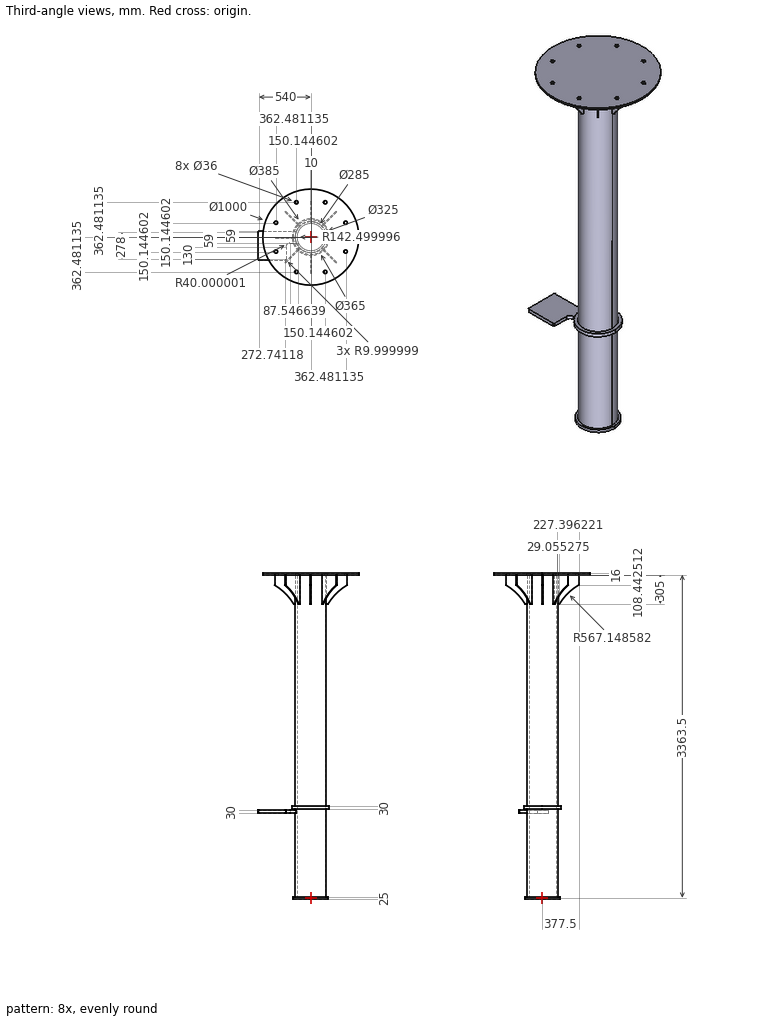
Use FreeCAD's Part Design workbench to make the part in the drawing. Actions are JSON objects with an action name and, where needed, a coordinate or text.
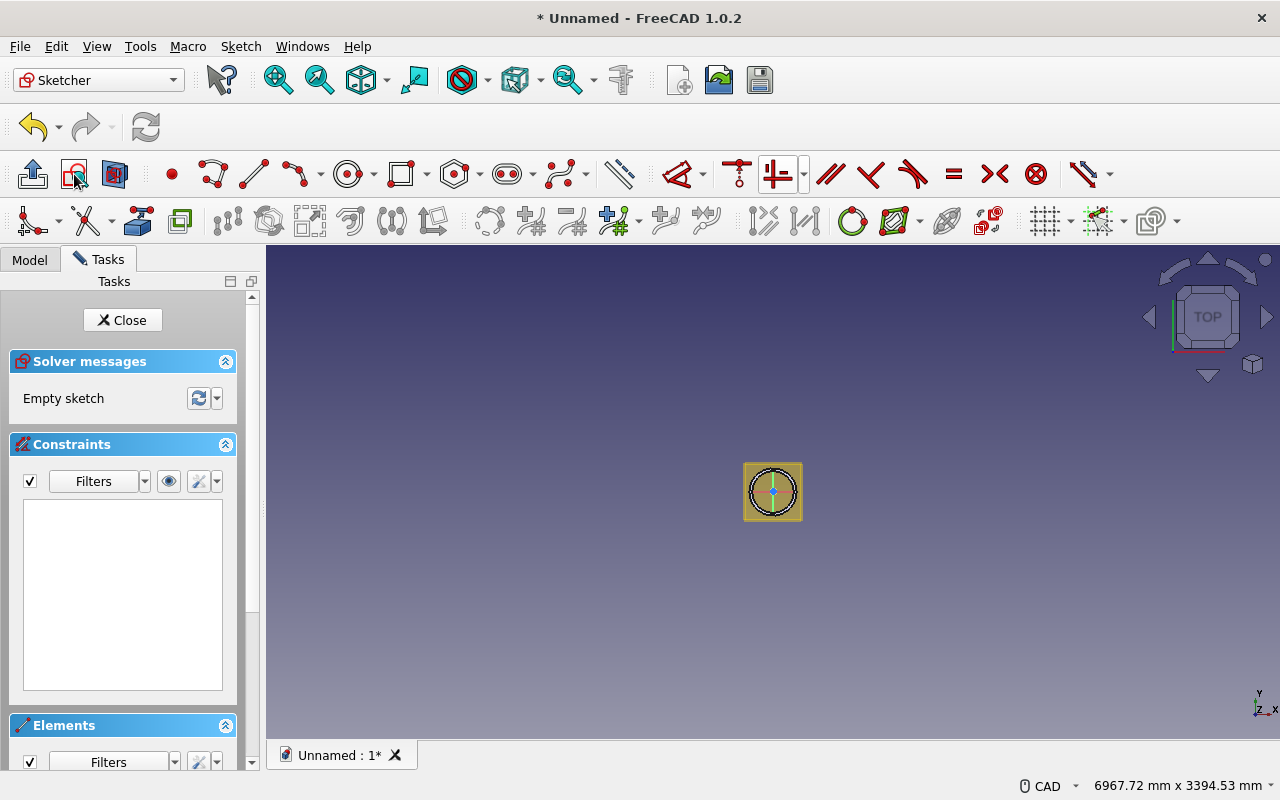
{"action": "key", "text": "q s"}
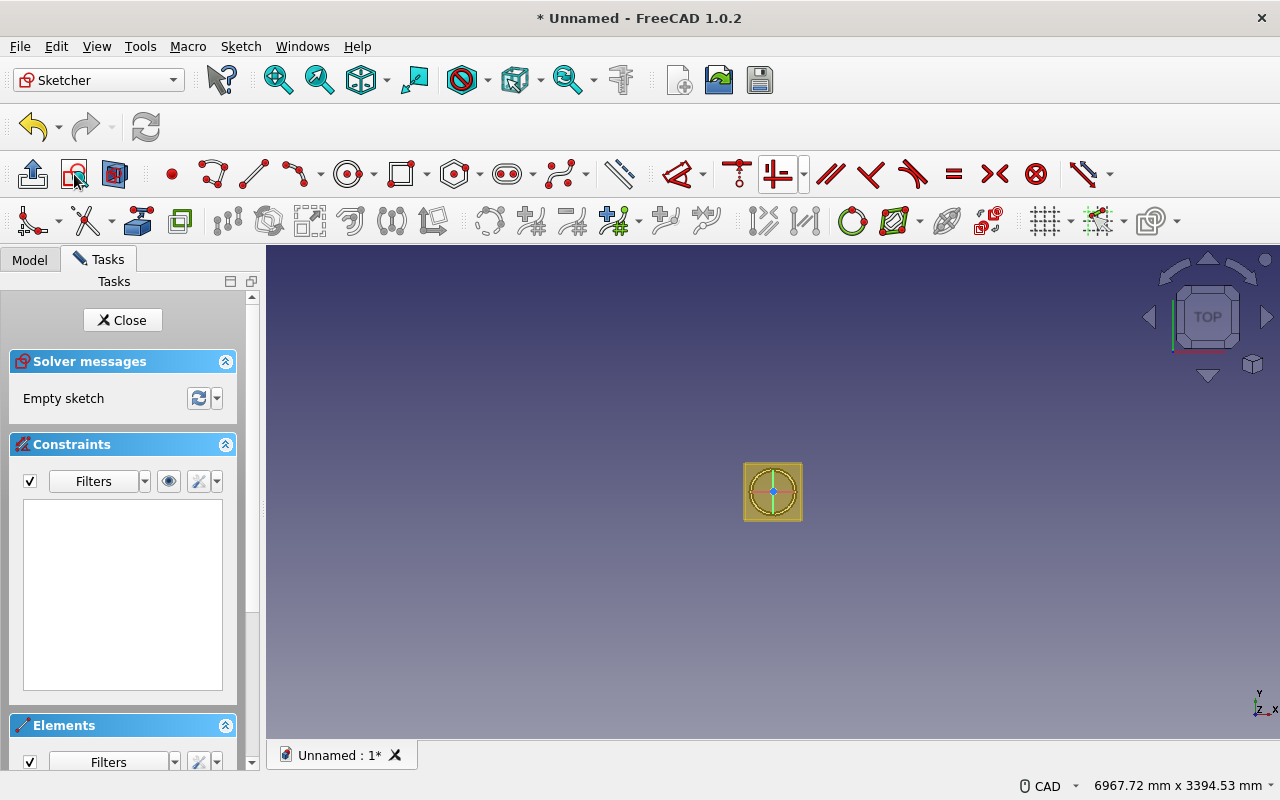
{"action": "scroll", "coordinate": [787, 492], "scroll_direction": "up", "scroll_amount": 9}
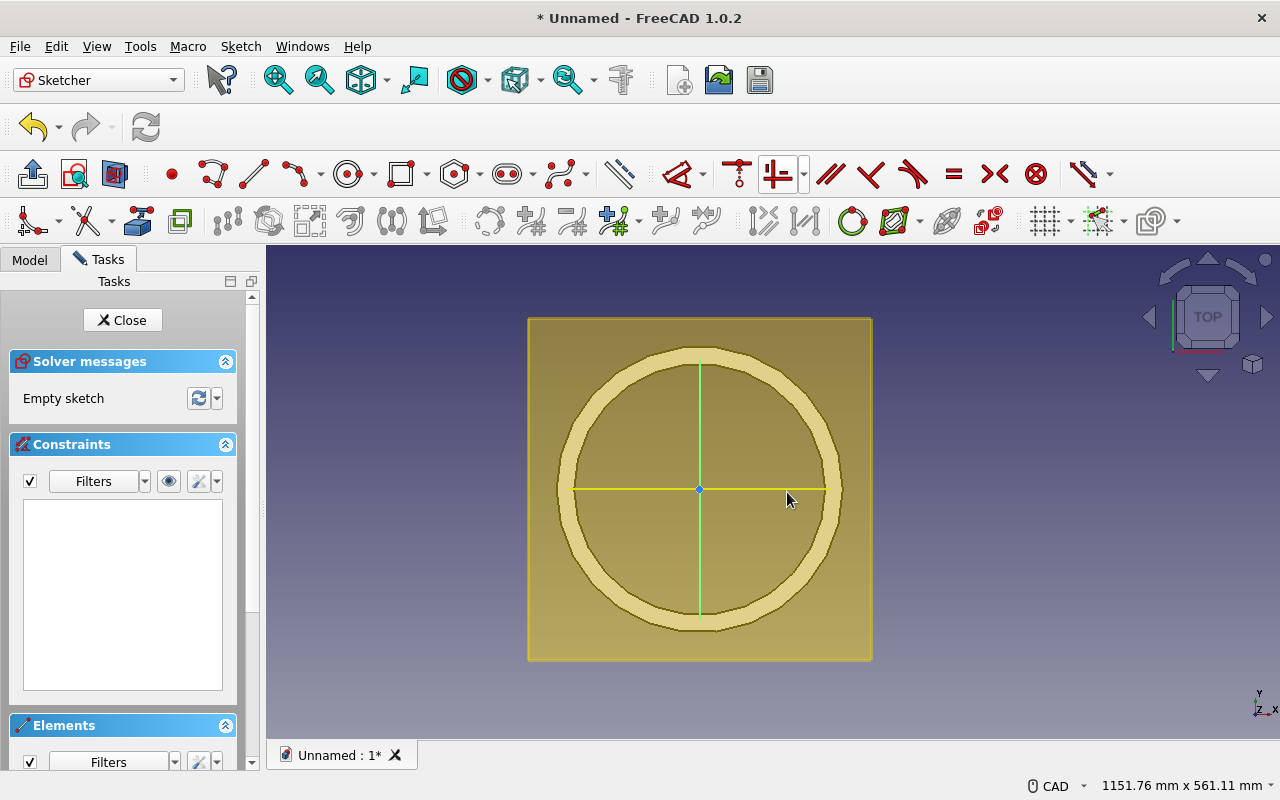
{"action": "left_click", "coordinate": [348, 174]}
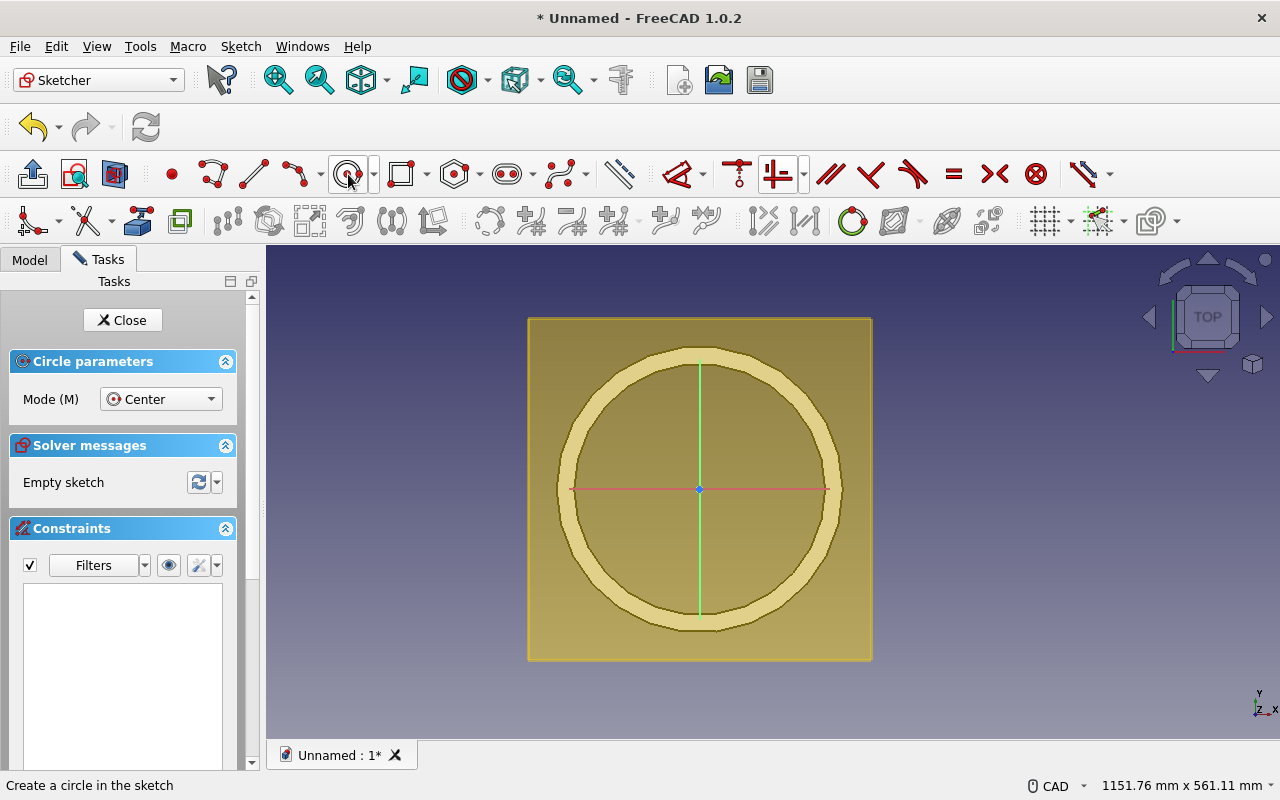
{"action": "left_click", "coordinate": [700, 489]}
{"action": "left_click", "coordinate": [820, 370]}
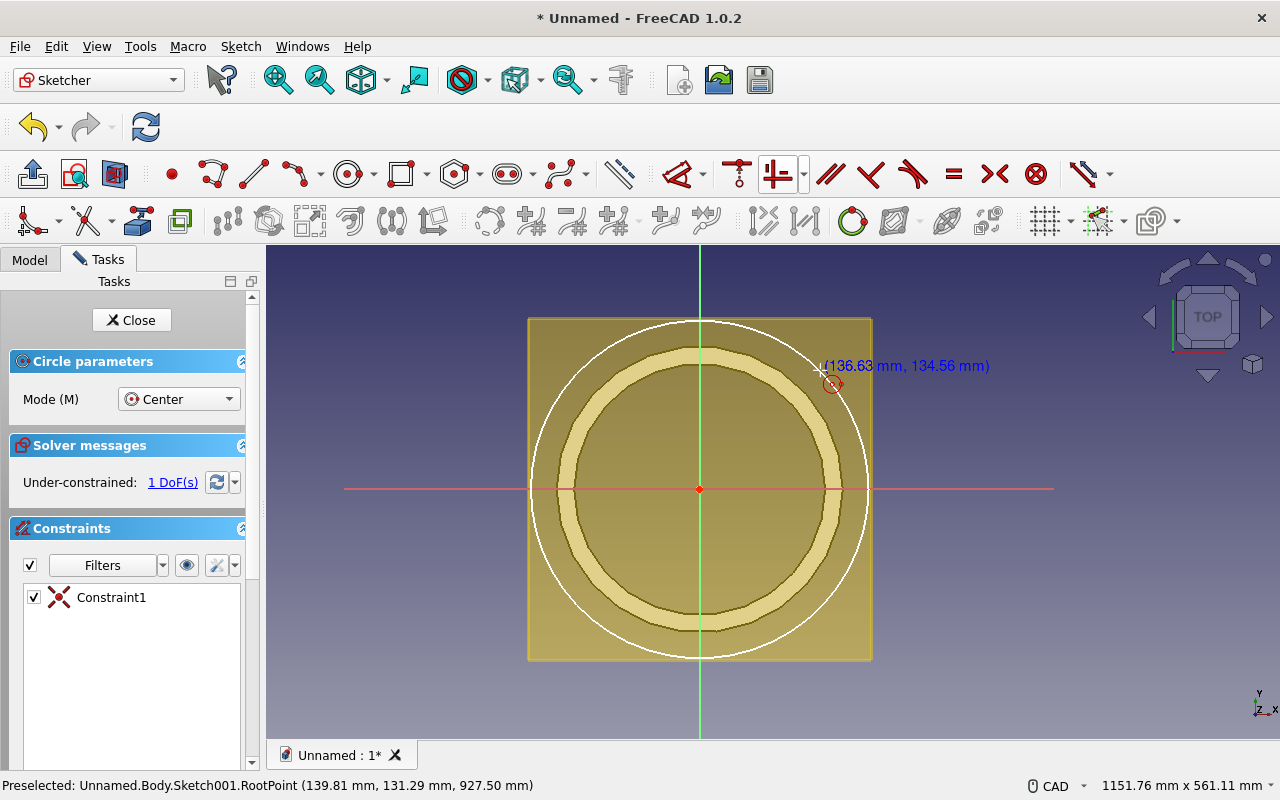
{"action": "left_click", "coordinate": [700, 489]}
{"action": "left_click", "coordinate": [801, 388]}
{"action": "key", "text": "Escape"}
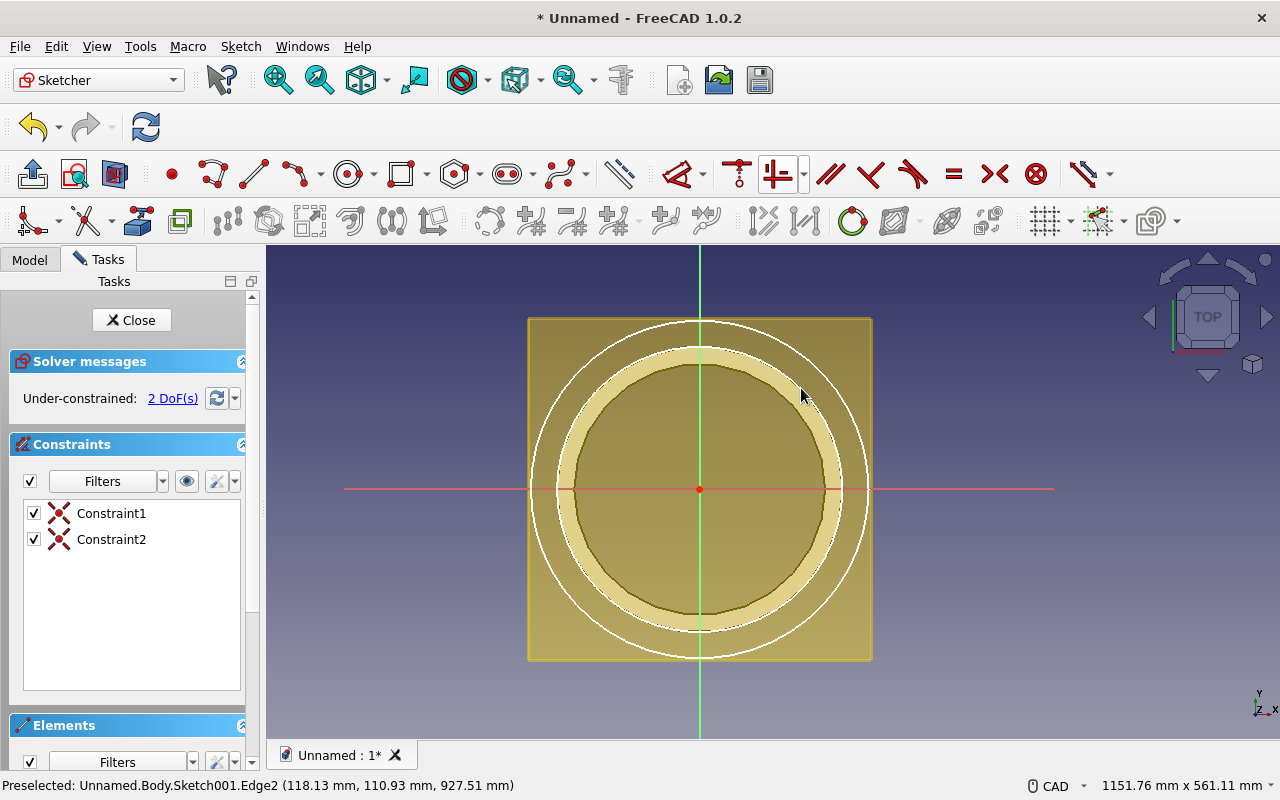
{"action": "left_click", "coordinate": [819, 370]}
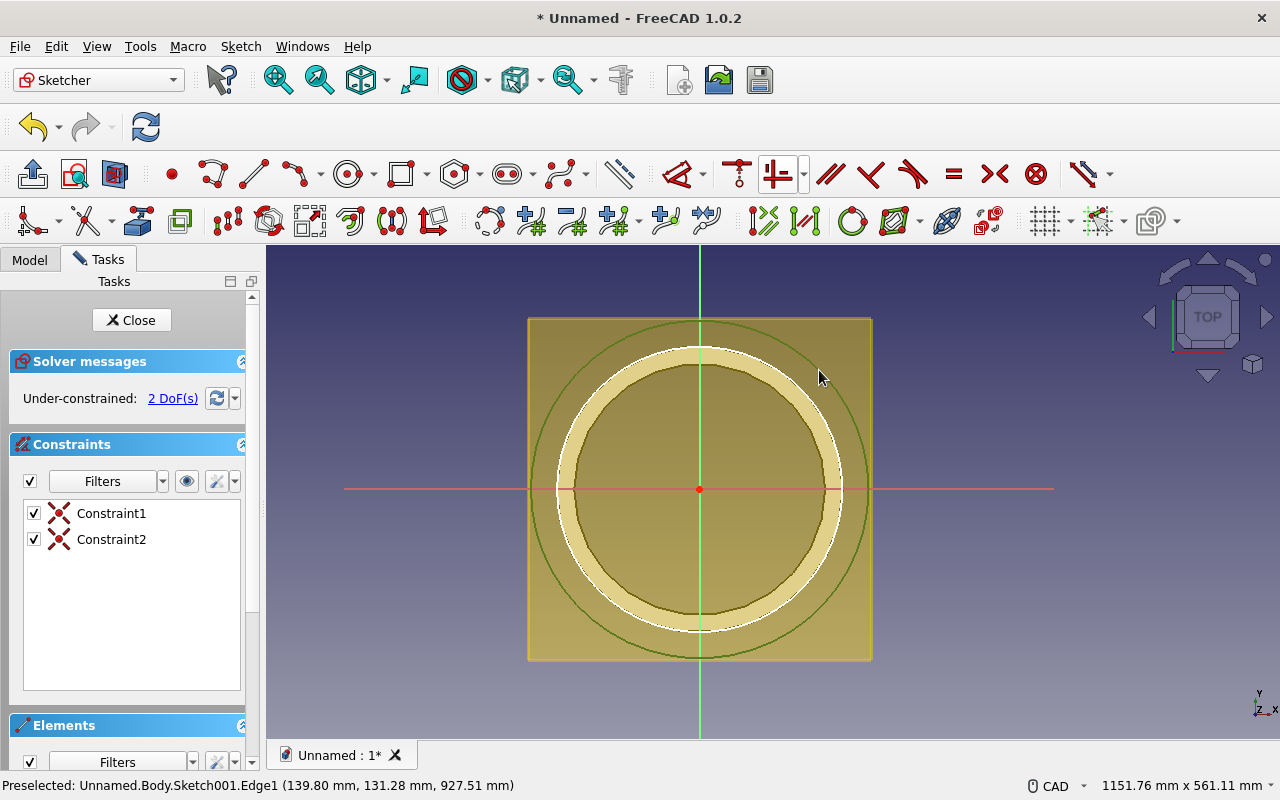
{"action": "key", "text": "k o"}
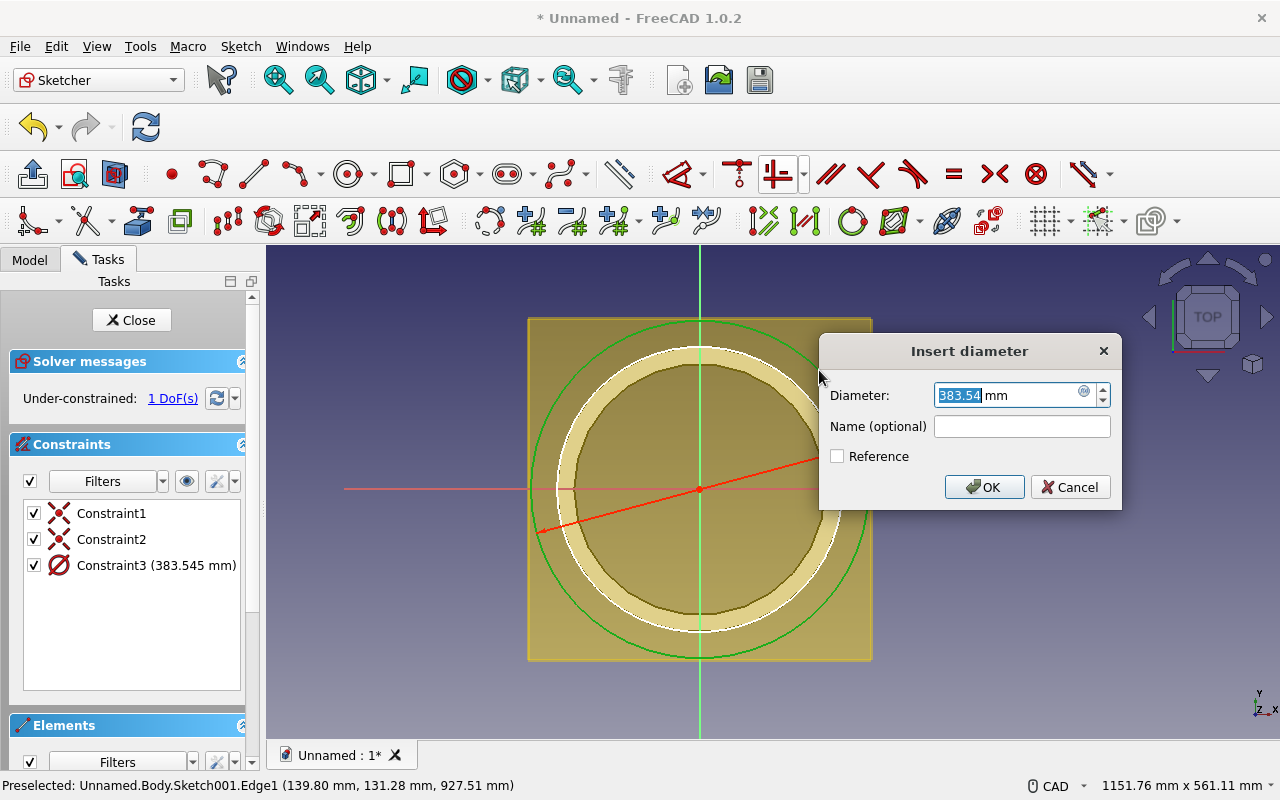
{"action": "type", "text": "385"}
{"action": "key", "text": "Return"}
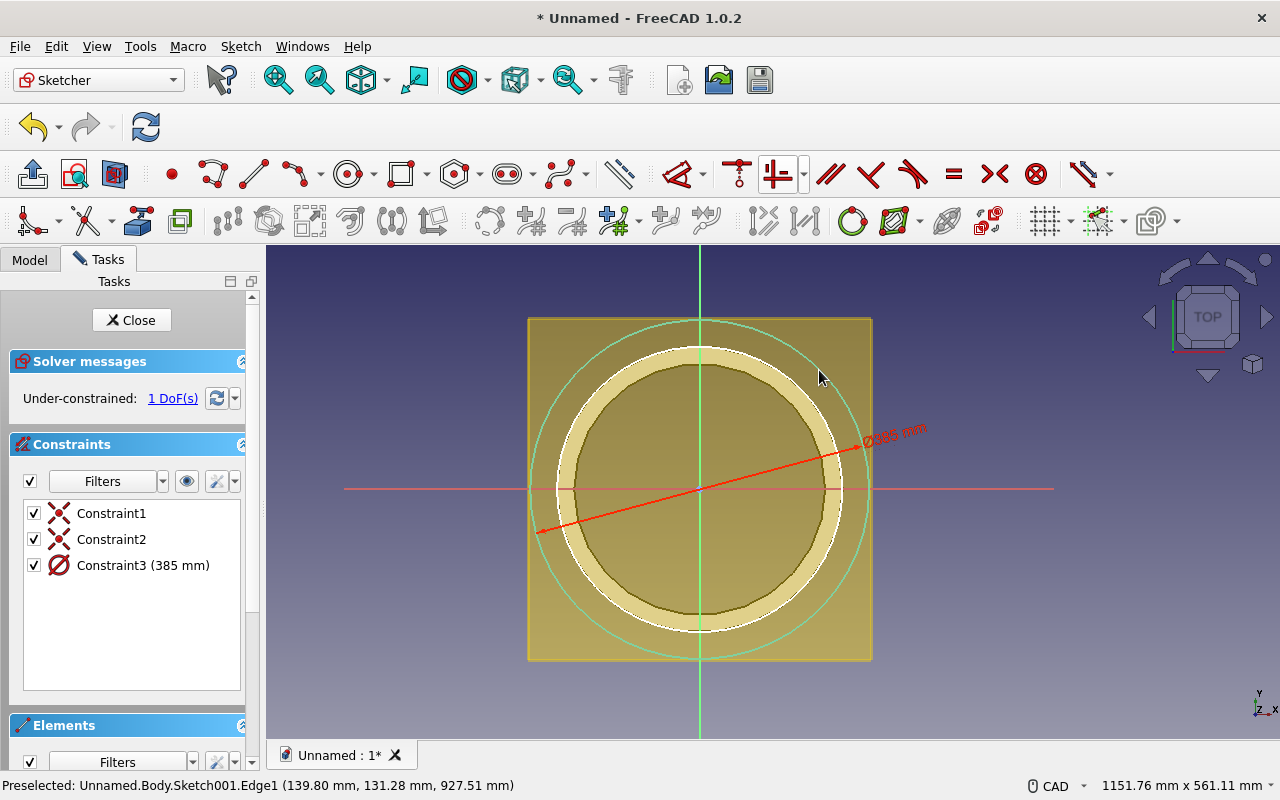
{"action": "left_click", "coordinate": [800, 388]}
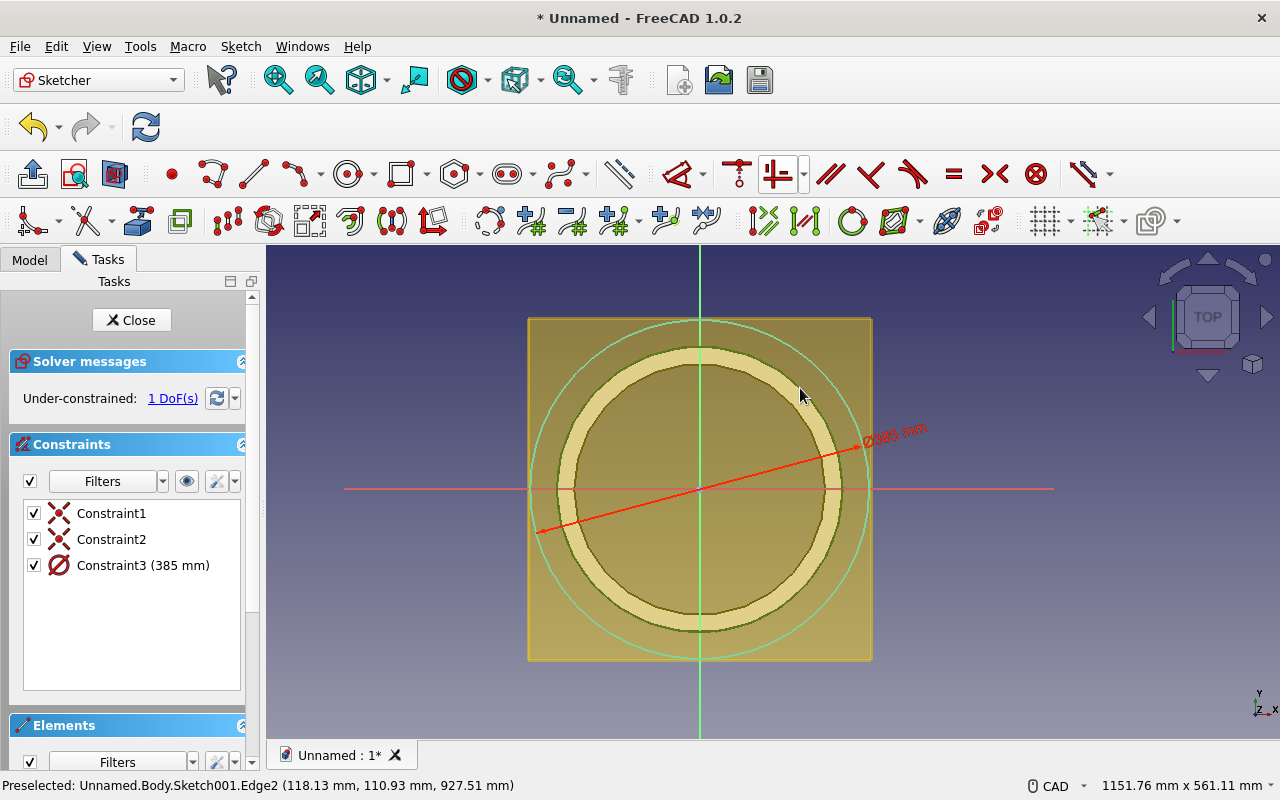
{"action": "key", "text": "k o"}